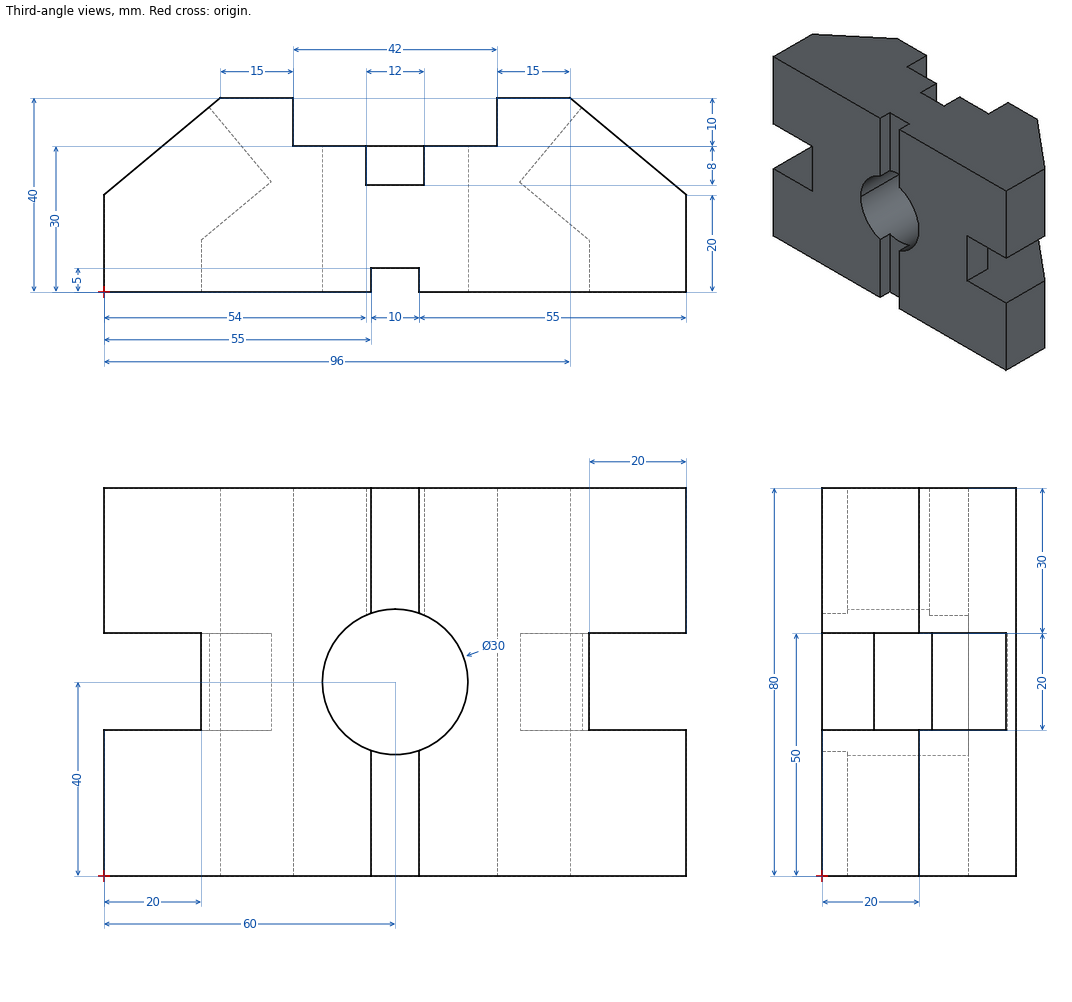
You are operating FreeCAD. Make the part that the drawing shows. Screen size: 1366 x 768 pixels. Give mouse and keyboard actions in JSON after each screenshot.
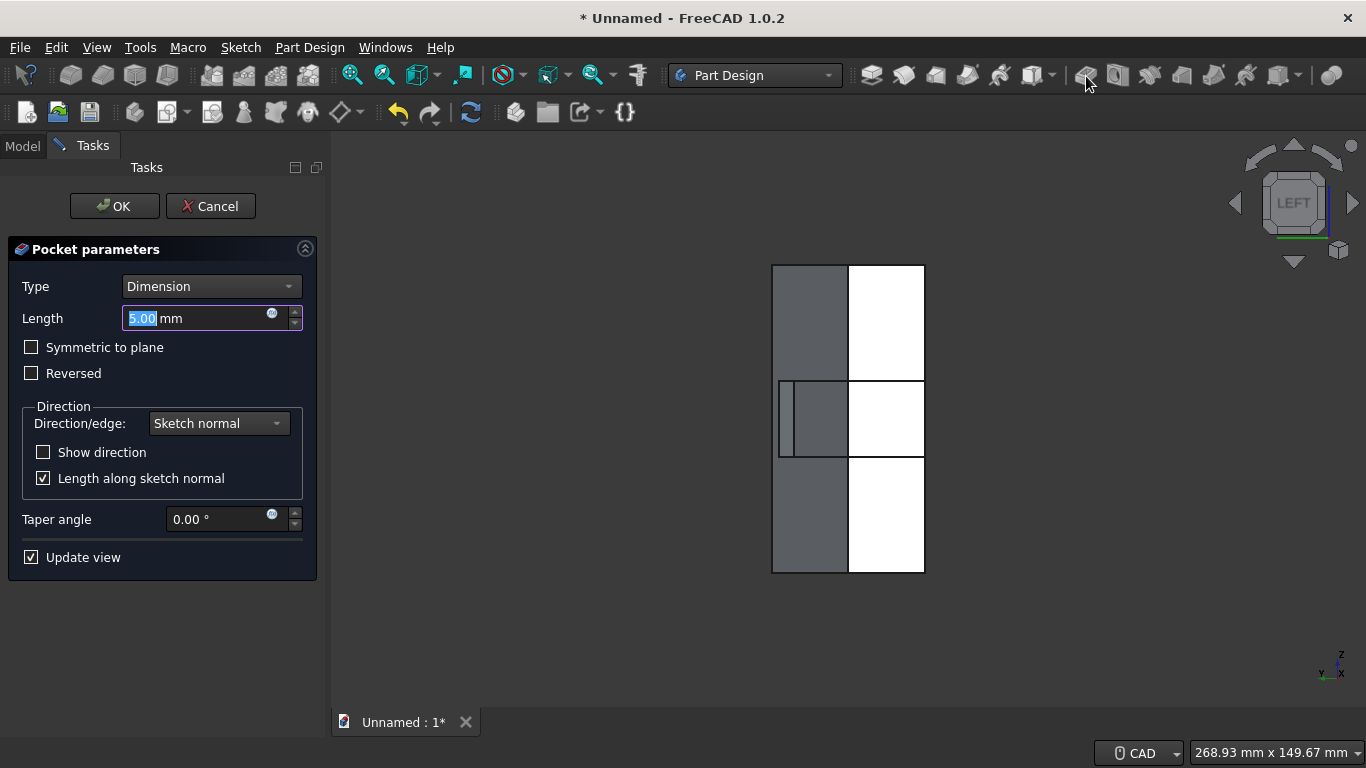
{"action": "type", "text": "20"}
{"action": "key", "text": "Tab"}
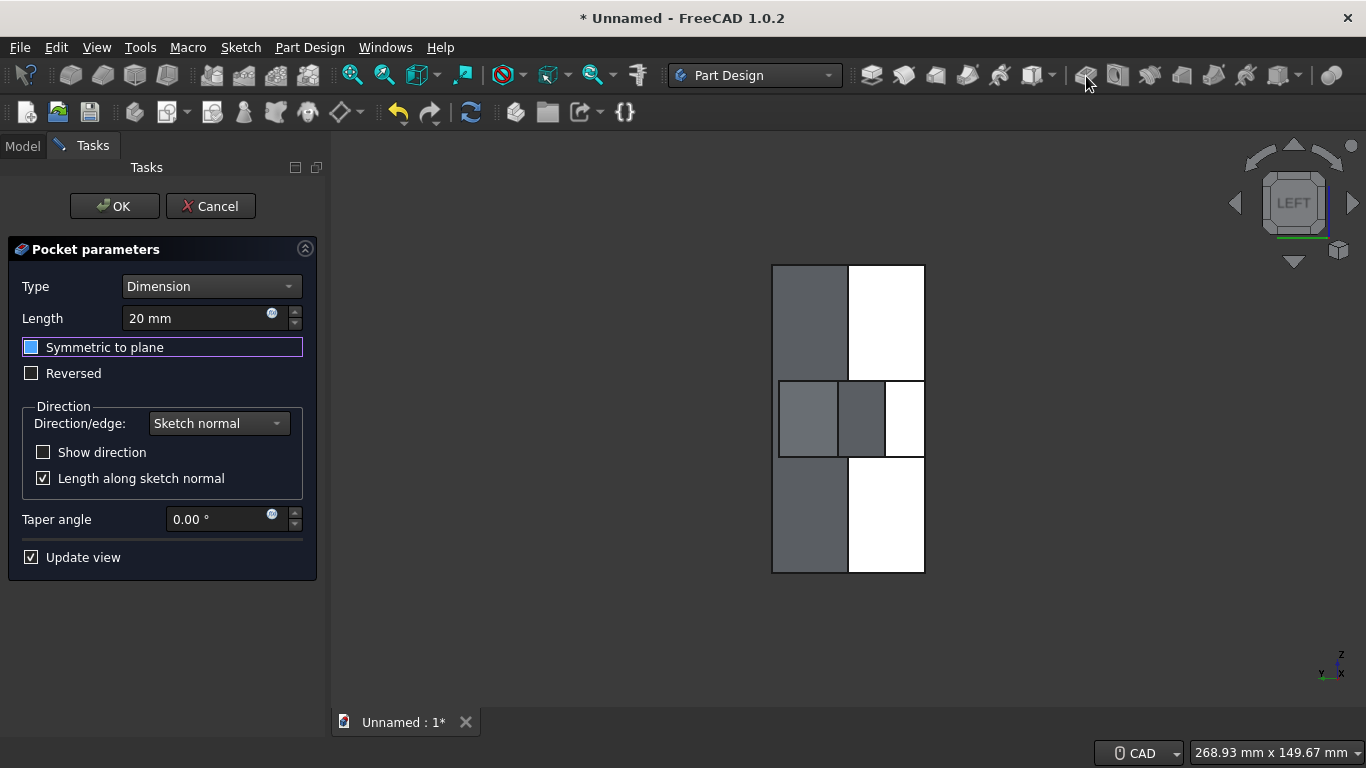
{"action": "left_click", "coordinate": [115, 206]}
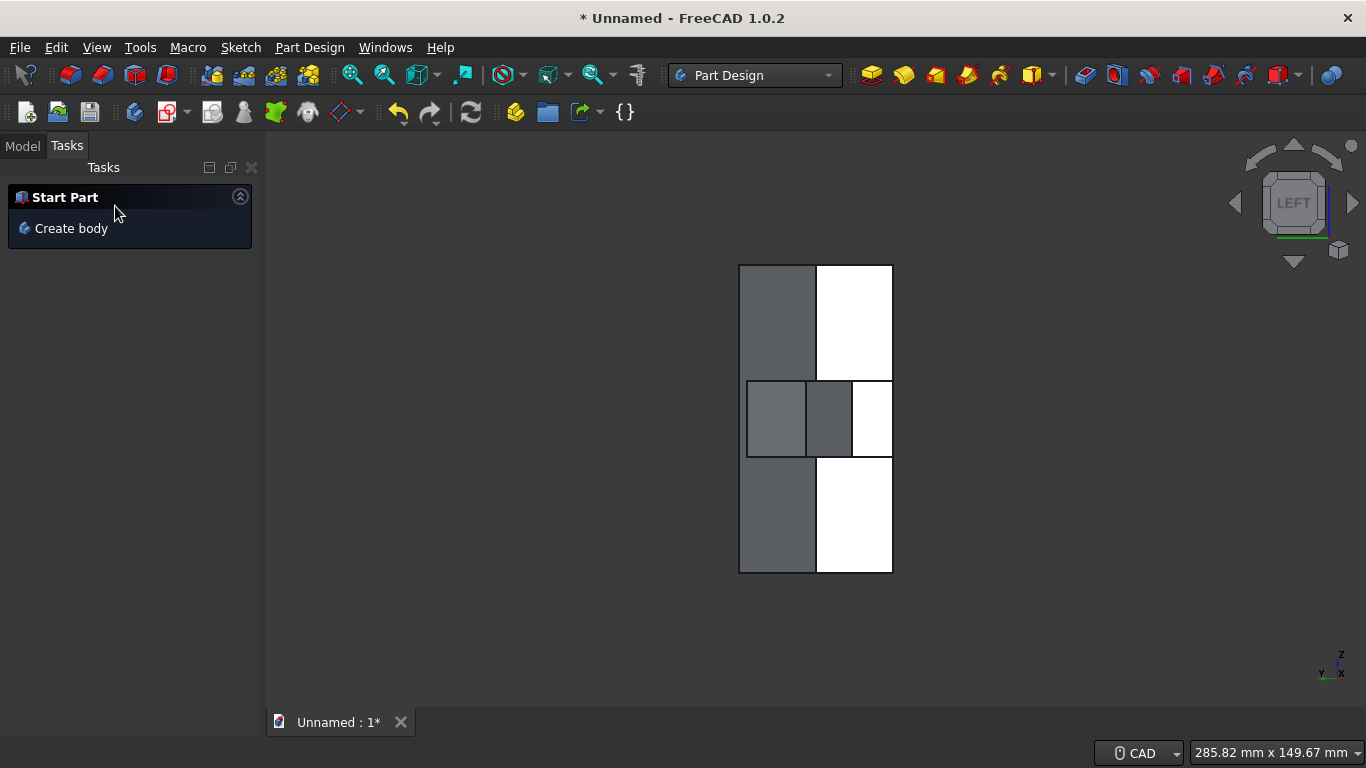
{"action": "key", "text": "0"}